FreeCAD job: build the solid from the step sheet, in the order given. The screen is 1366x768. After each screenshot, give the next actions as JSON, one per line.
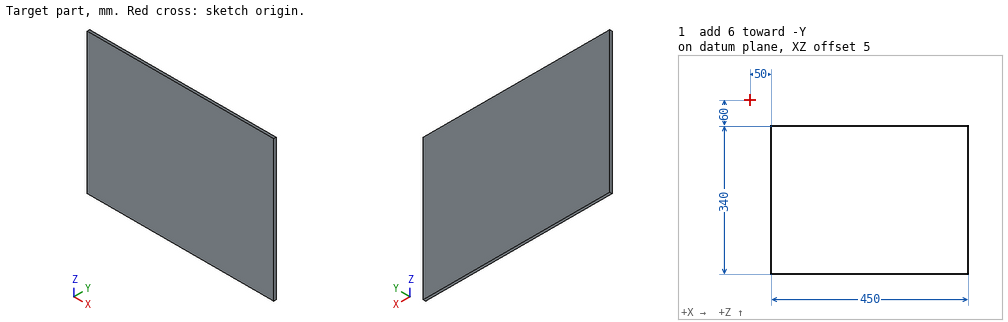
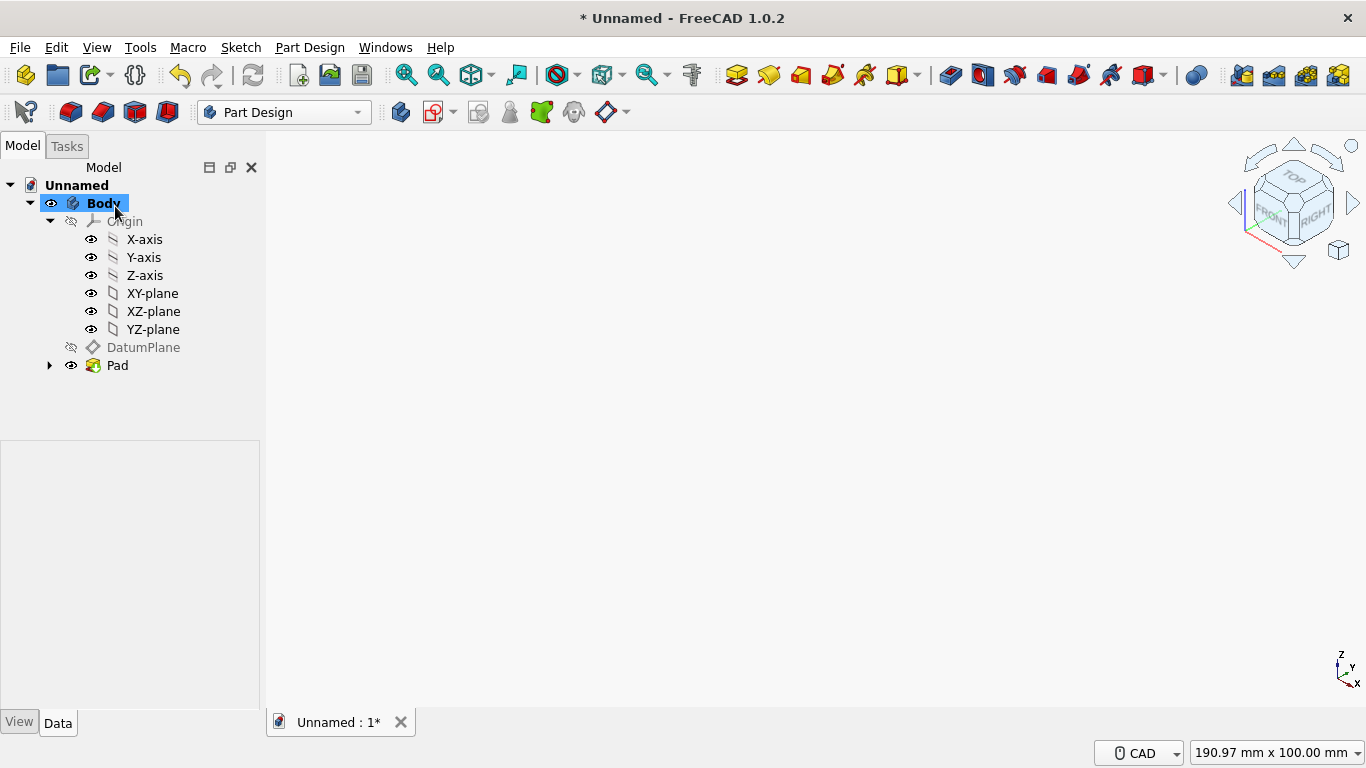
{"action": "left_click", "coordinate": [408, 76]}